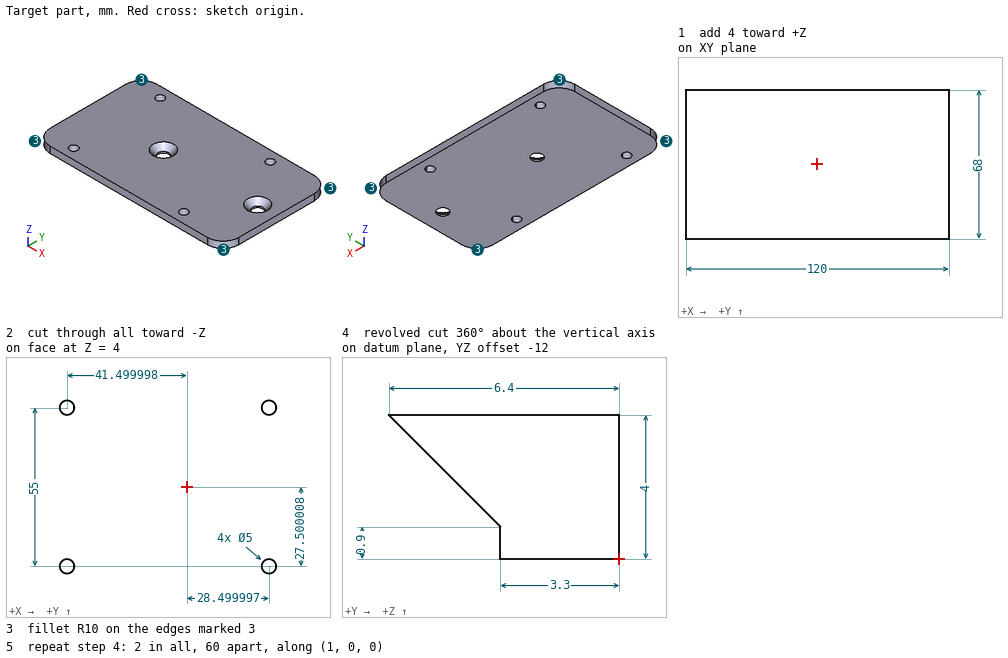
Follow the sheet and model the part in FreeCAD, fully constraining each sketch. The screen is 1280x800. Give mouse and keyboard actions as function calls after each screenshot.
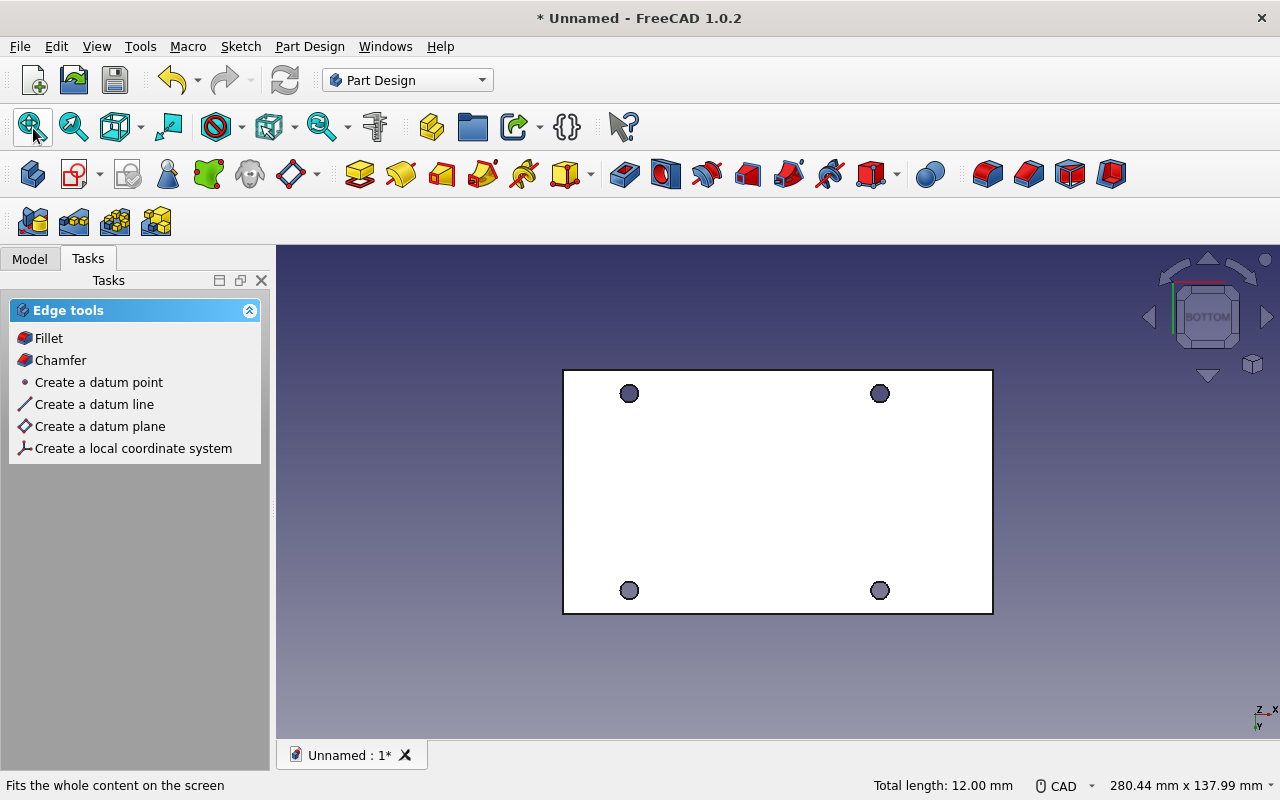
scroll(563, 613, up, 6)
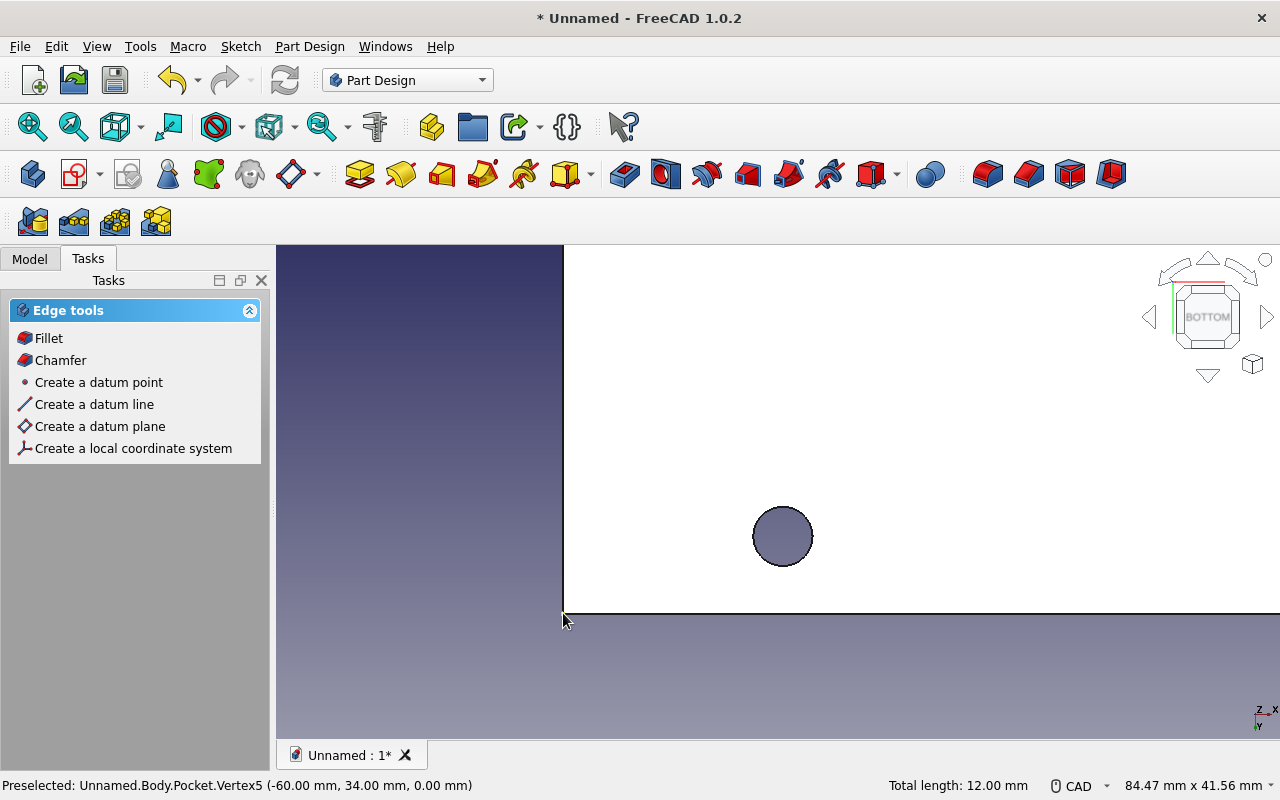
key(v)
key(f)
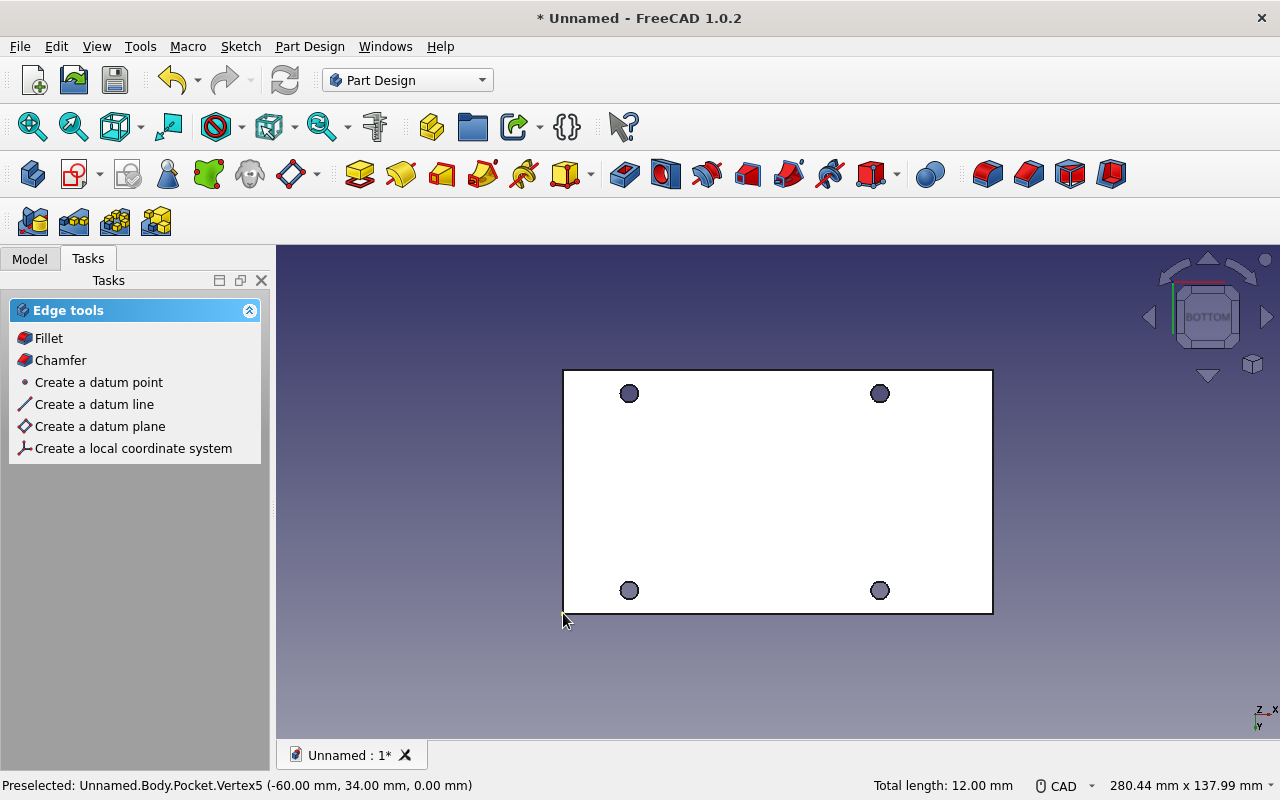
key(4)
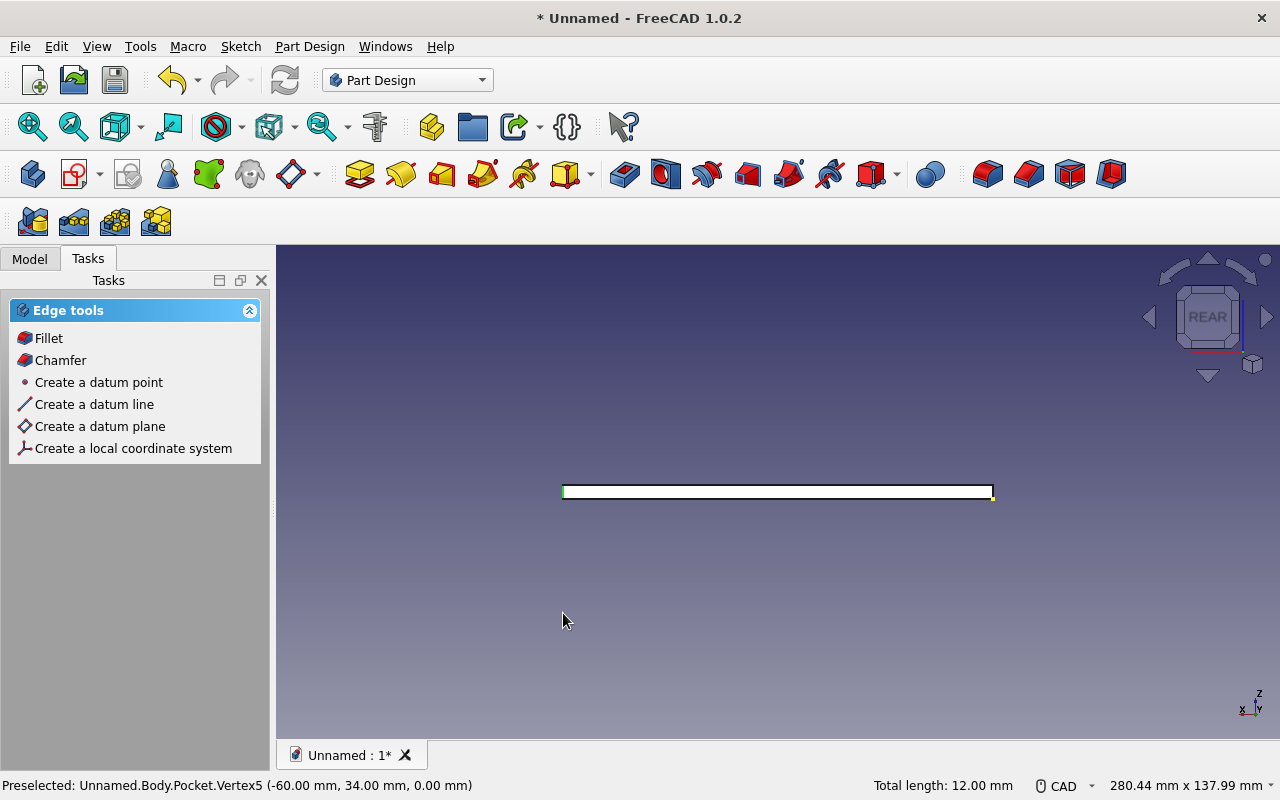
click(33, 128)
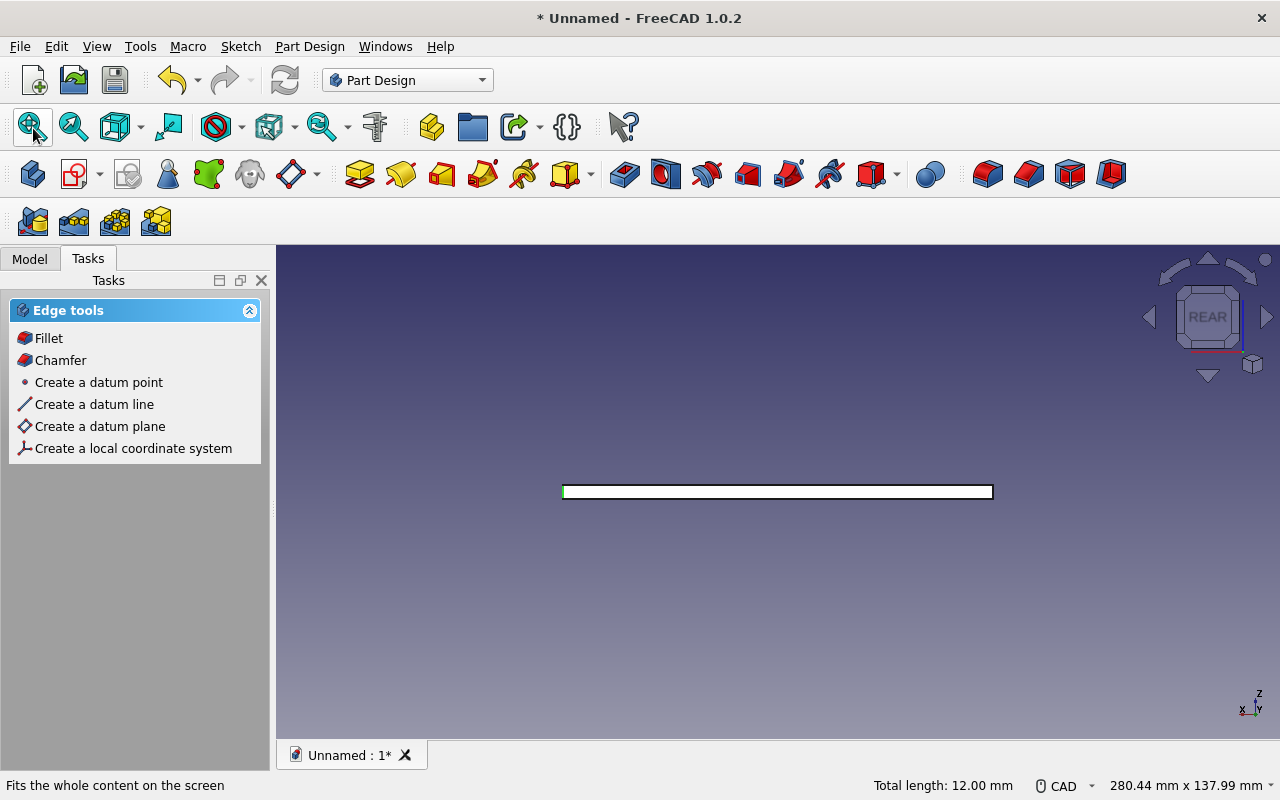
click(993, 491, ctrl)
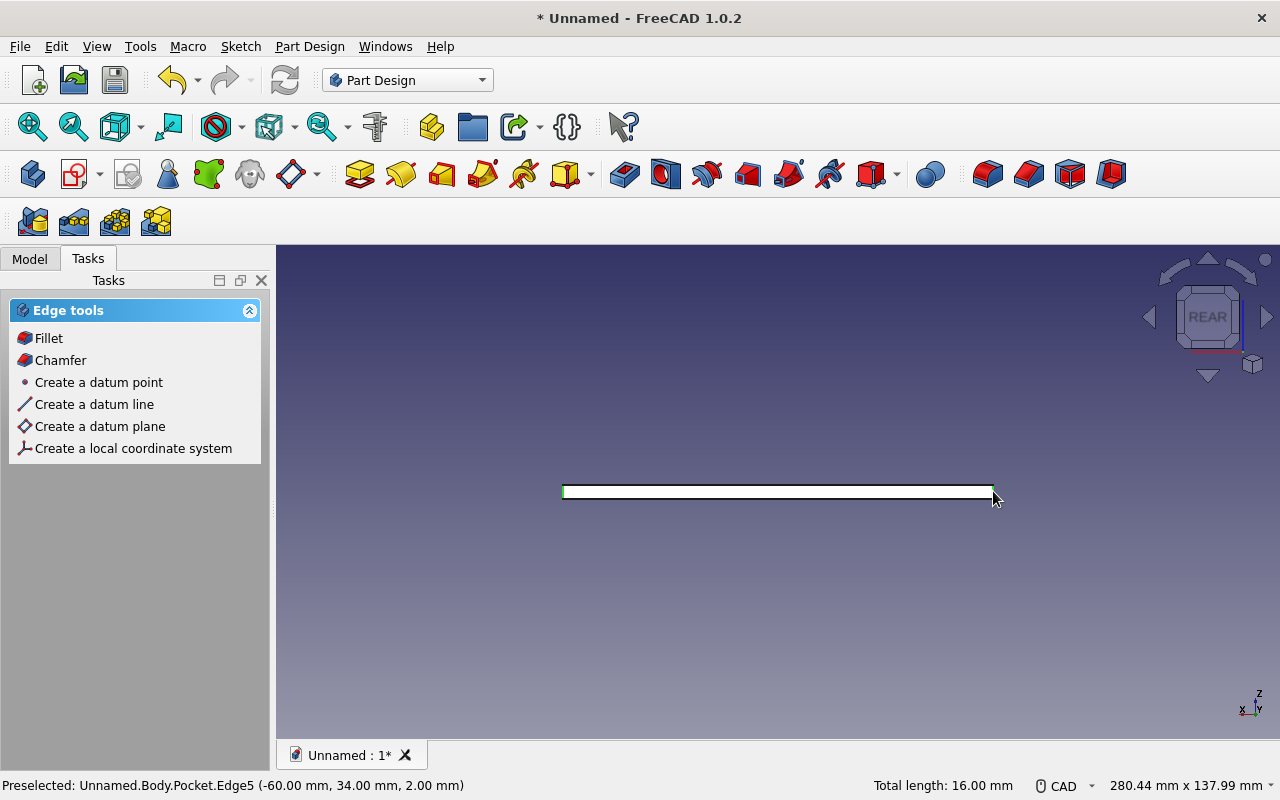
click(988, 174)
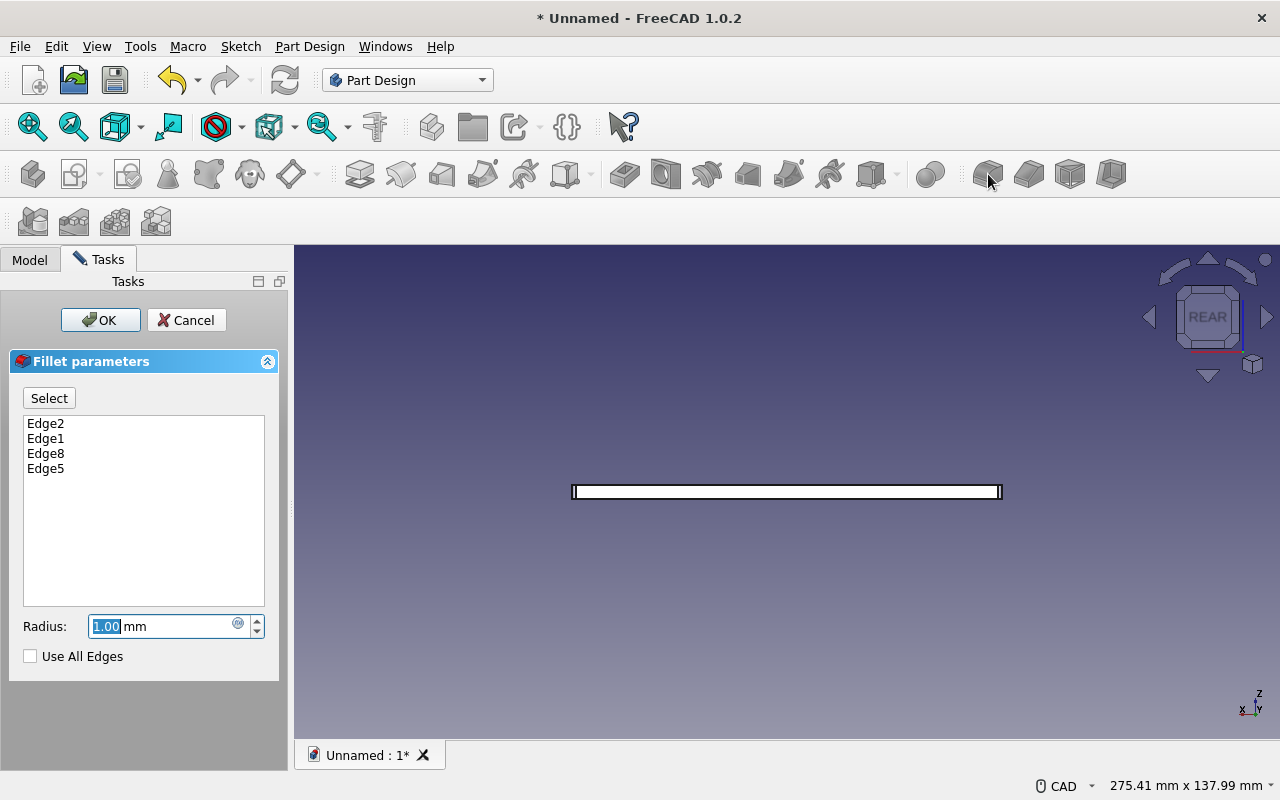
text(10)
key(Tab)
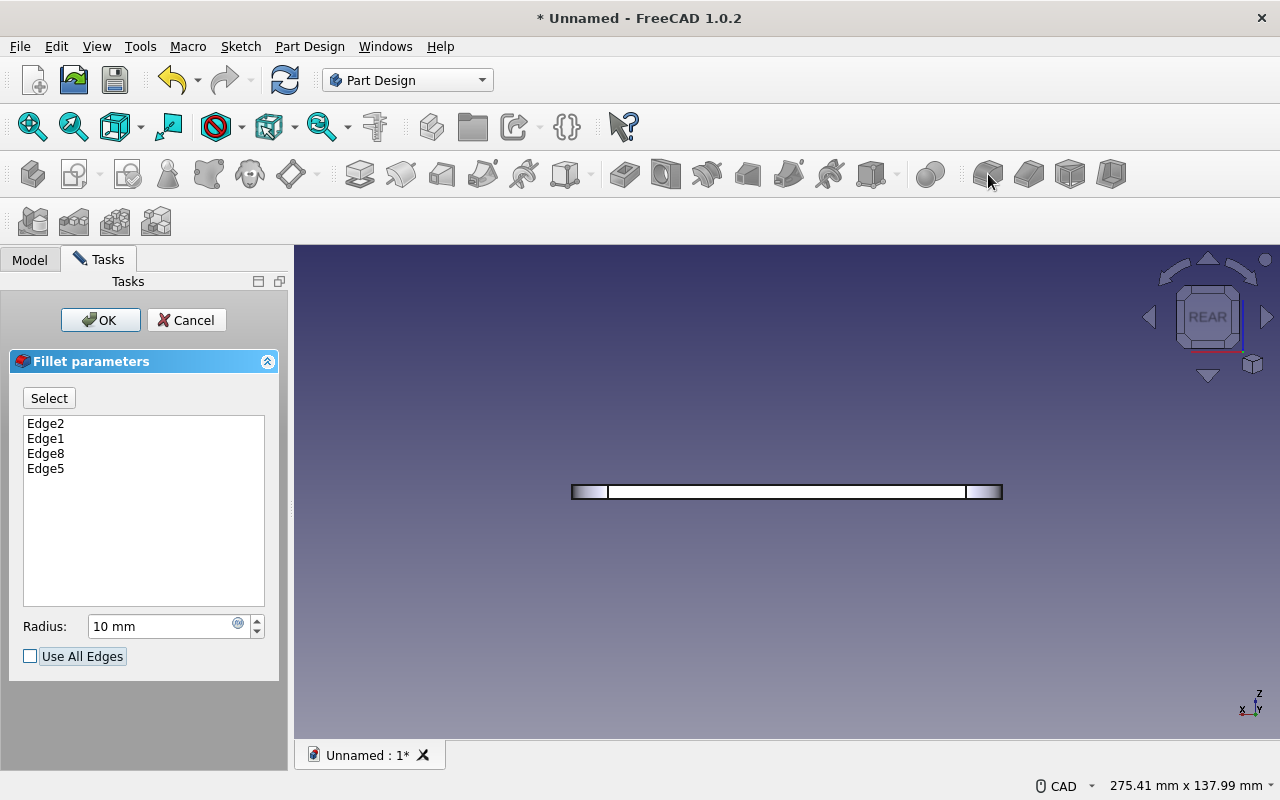
click(101, 320)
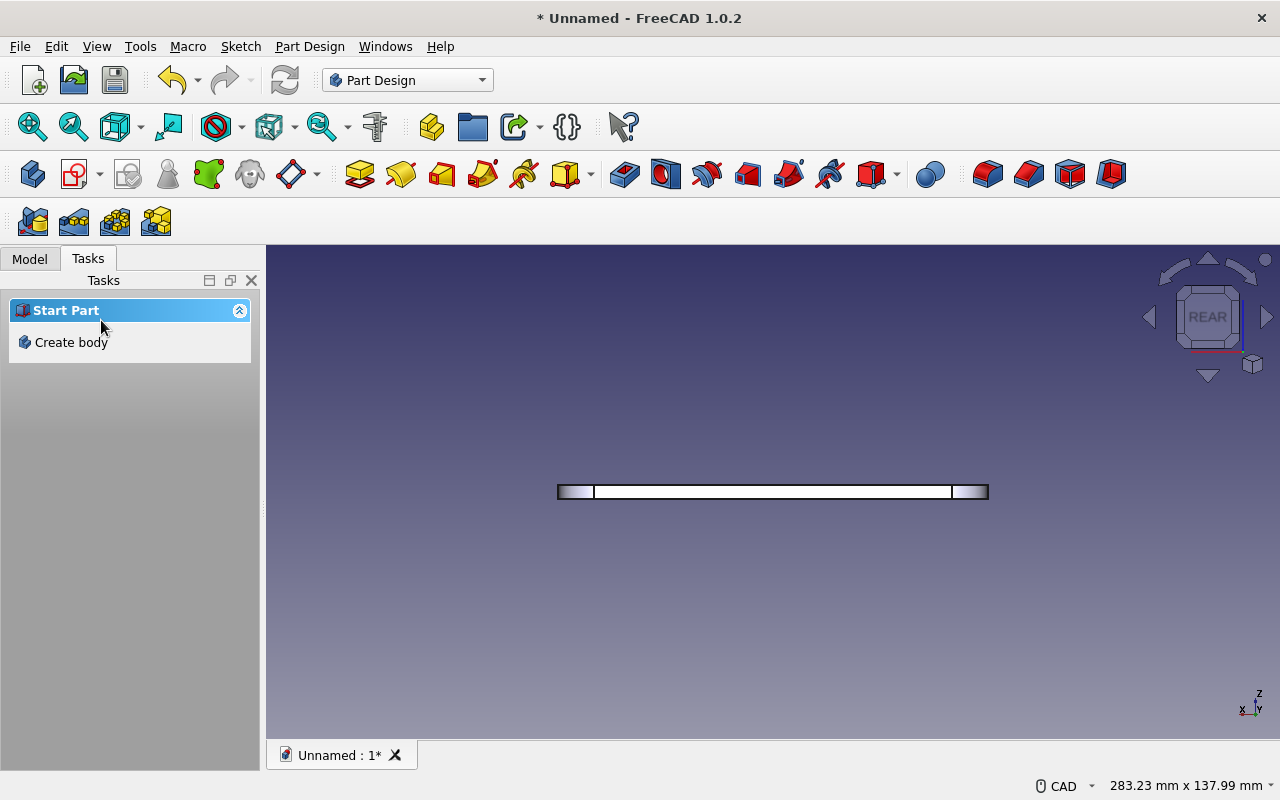
key(v)
key(f)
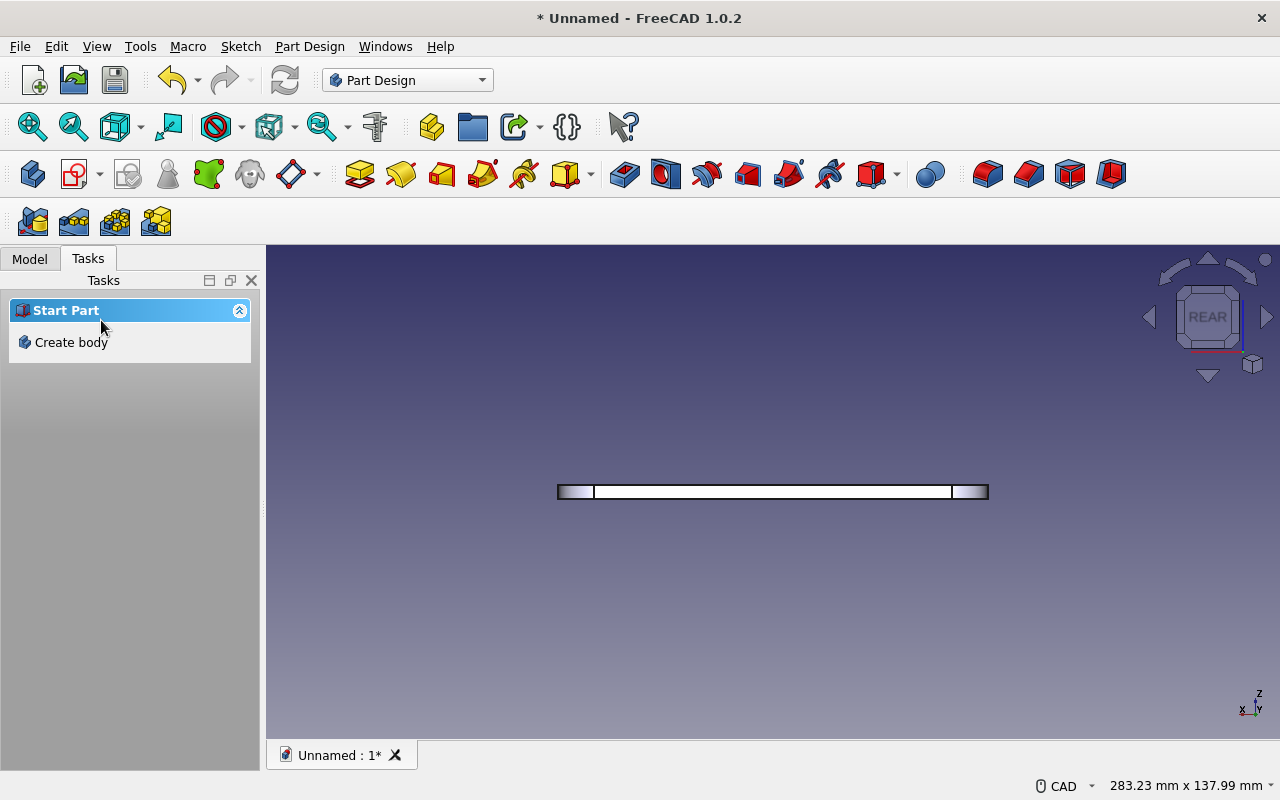
click(30, 258)